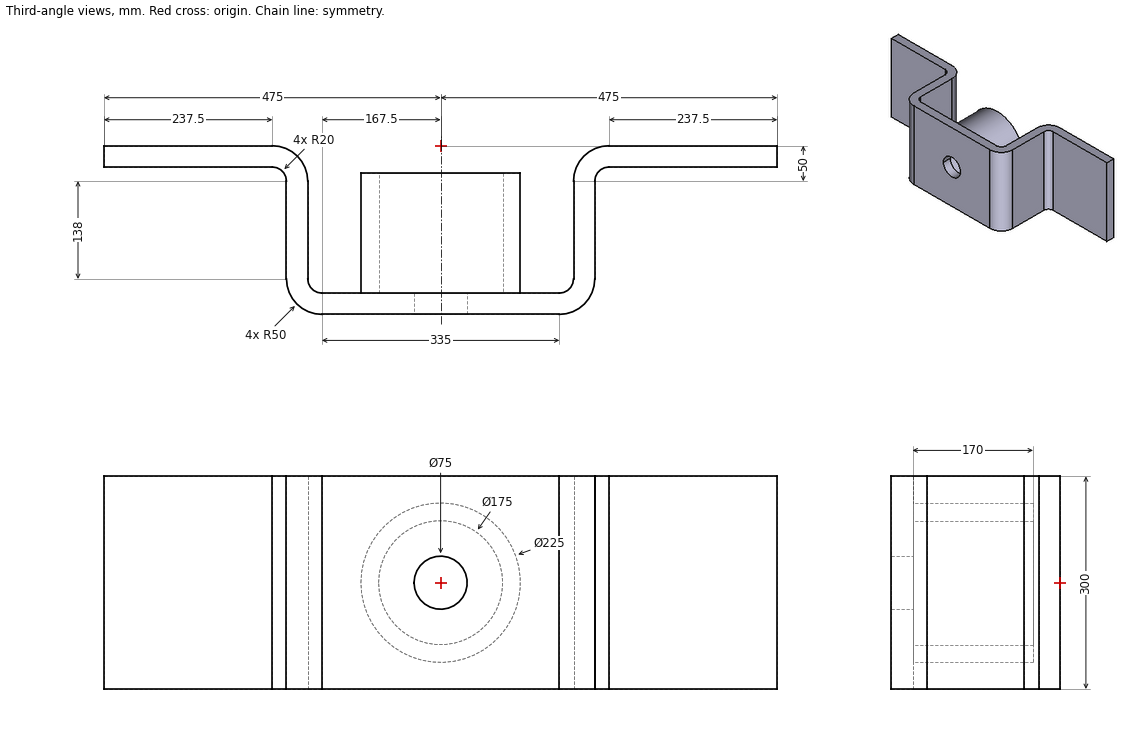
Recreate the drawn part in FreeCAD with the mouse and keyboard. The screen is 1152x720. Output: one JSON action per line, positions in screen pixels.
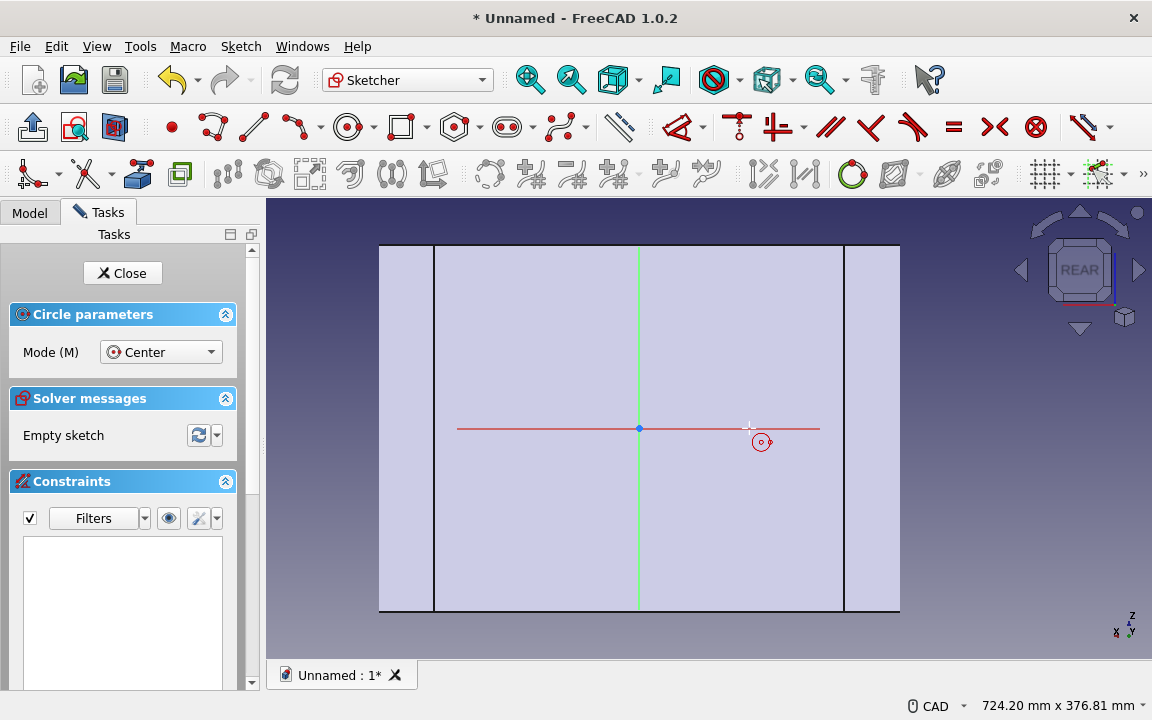
{"action": "left_click", "coordinate": [639, 428]}
{"action": "left_click", "coordinate": [737, 331]}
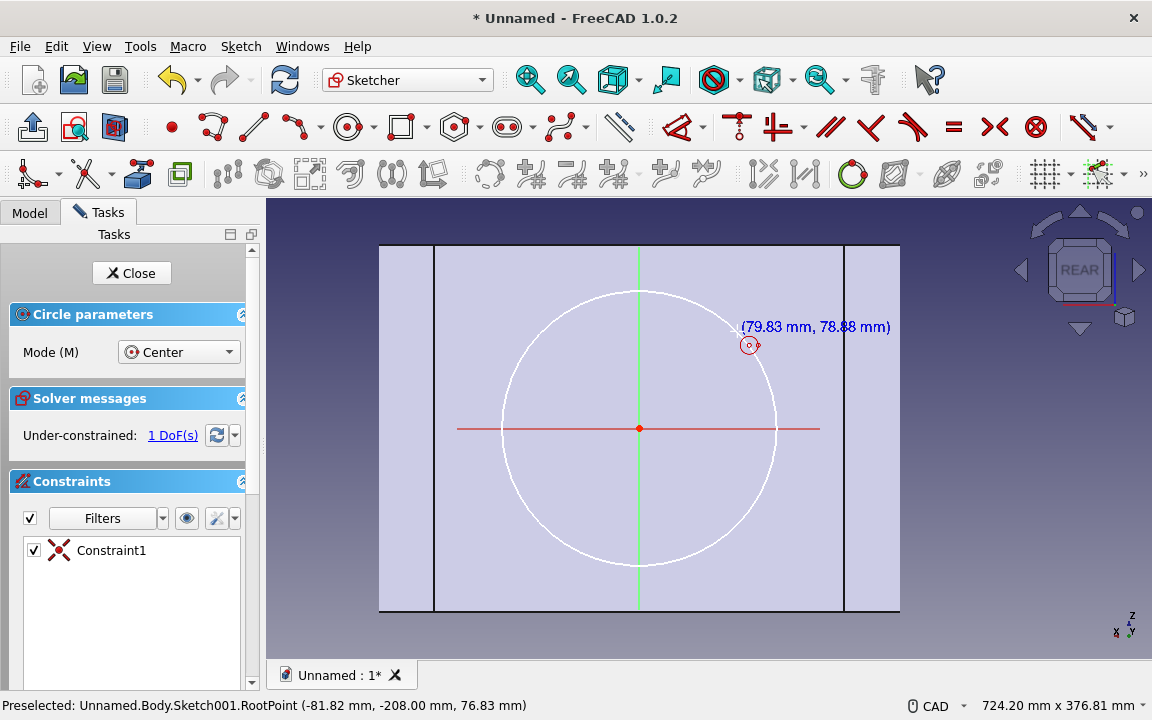
{"action": "left_click", "coordinate": [639, 428]}
{"action": "left_click", "coordinate": [715, 353]}
{"action": "key", "text": "Escape"}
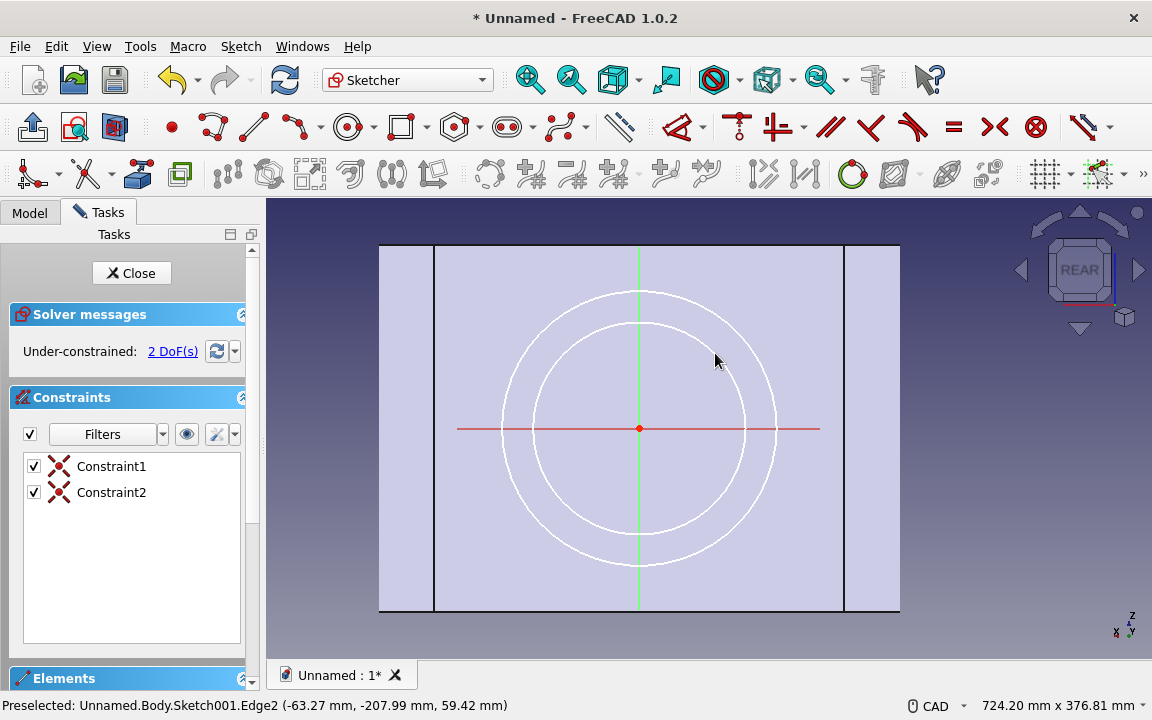
{"action": "key", "text": "d"}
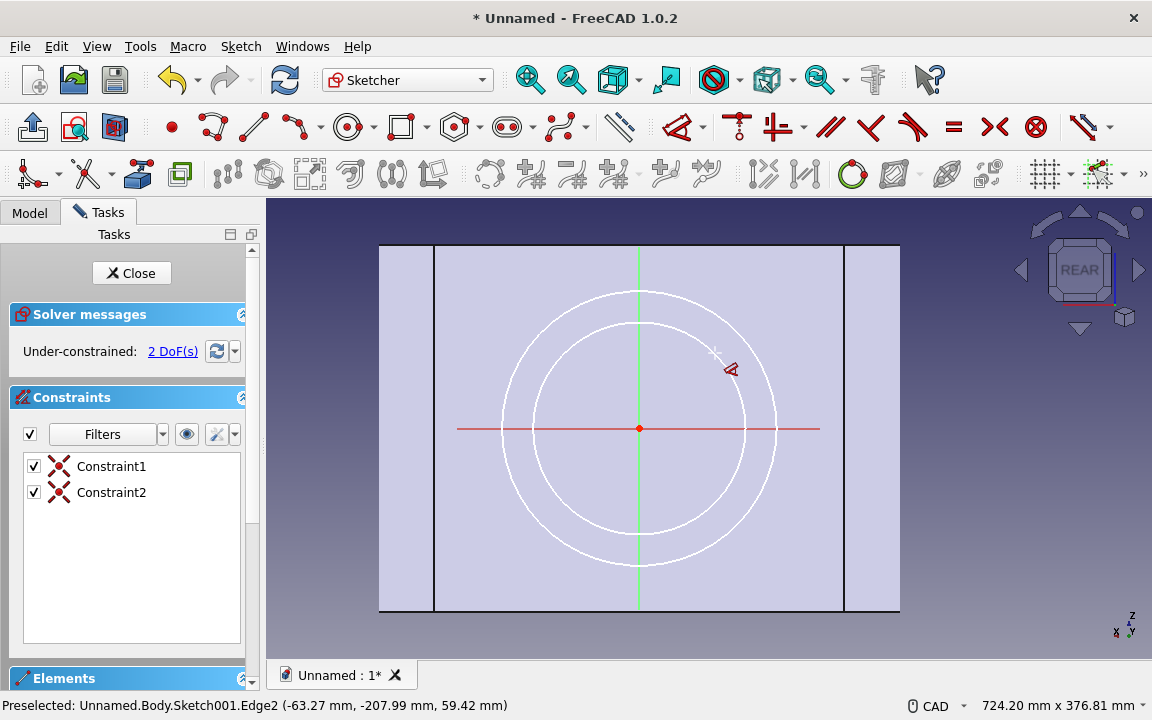
{"action": "left_click", "coordinate": [736, 331]}
{"action": "left_click", "coordinate": [759, 308]}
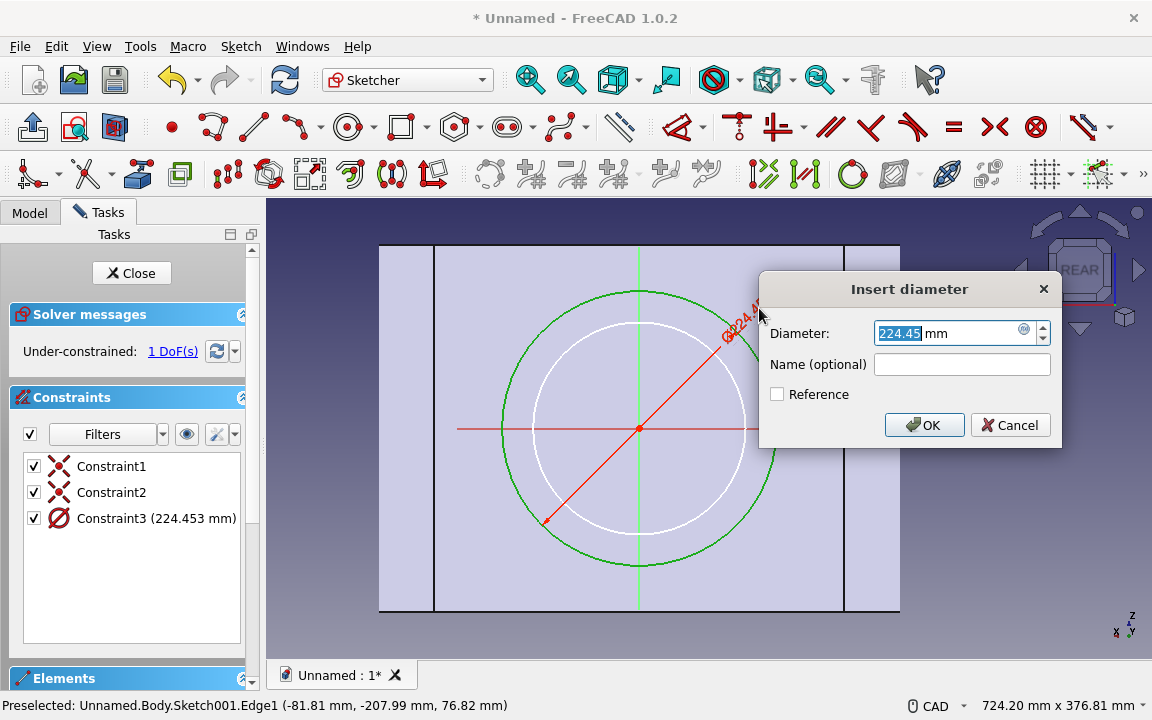
{"action": "type", "text": "225"}
{"action": "key", "text": "Return"}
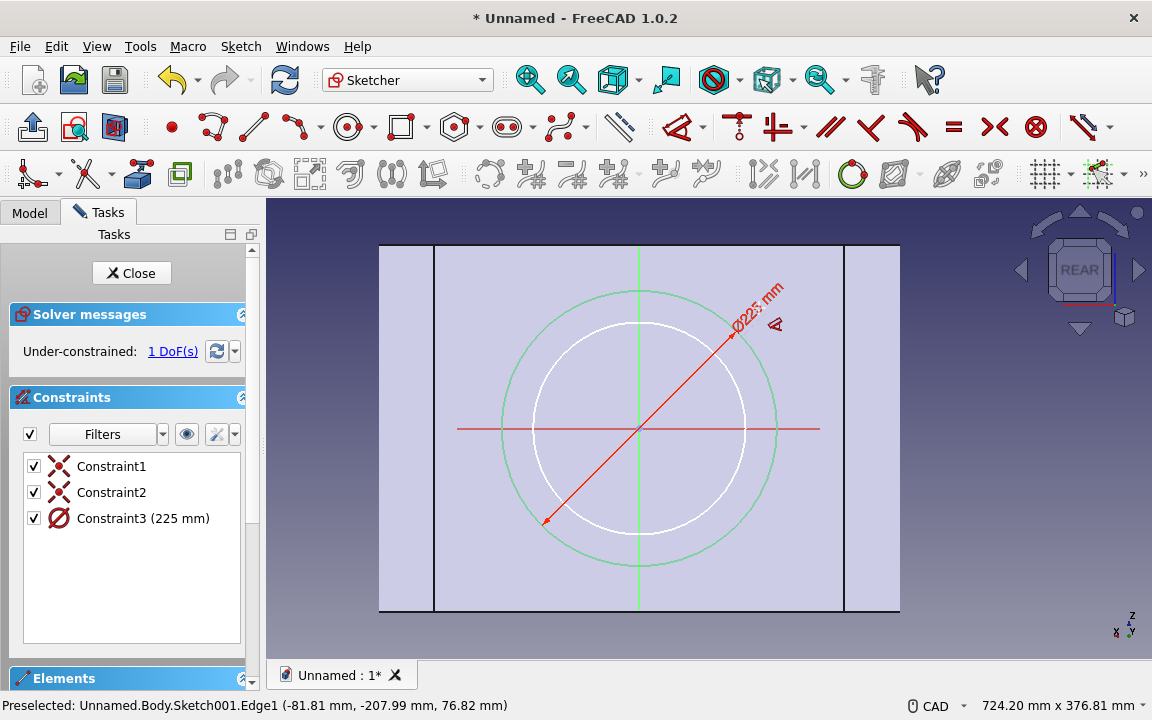
{"action": "left_click", "coordinate": [714, 353]}
{"action": "left_click", "coordinate": [794, 382]}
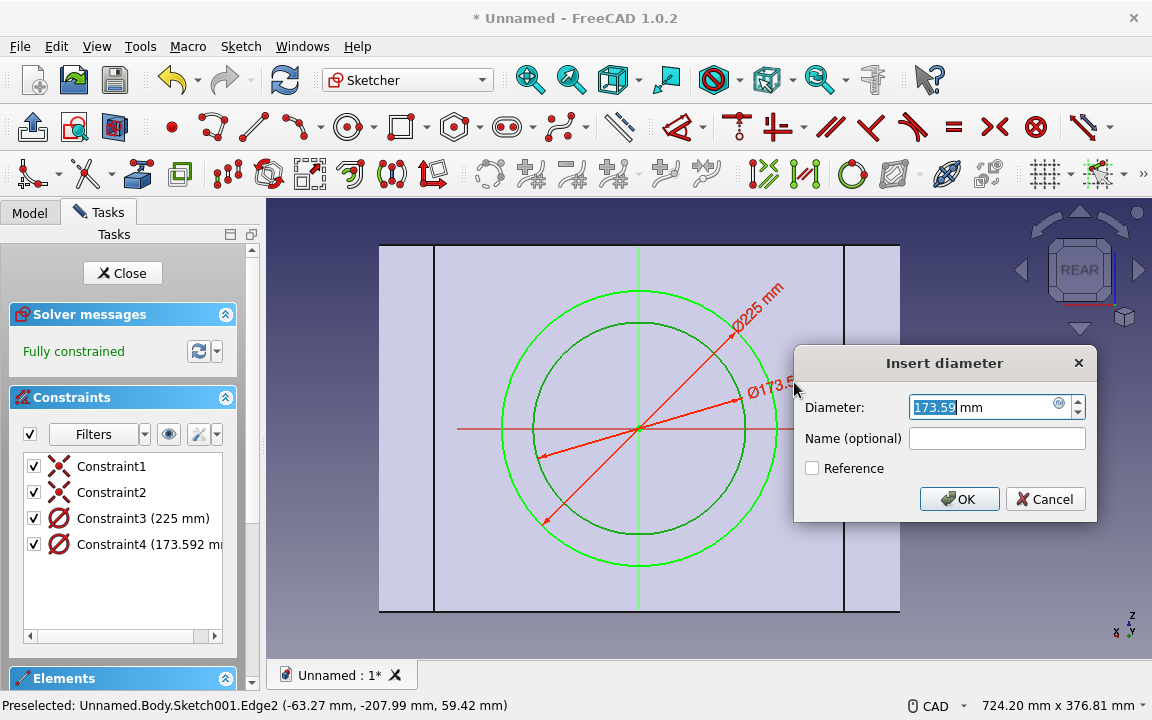
{"action": "type", "text": "175"}
{"action": "key", "text": "Return"}
{"action": "key", "text": "Escape"}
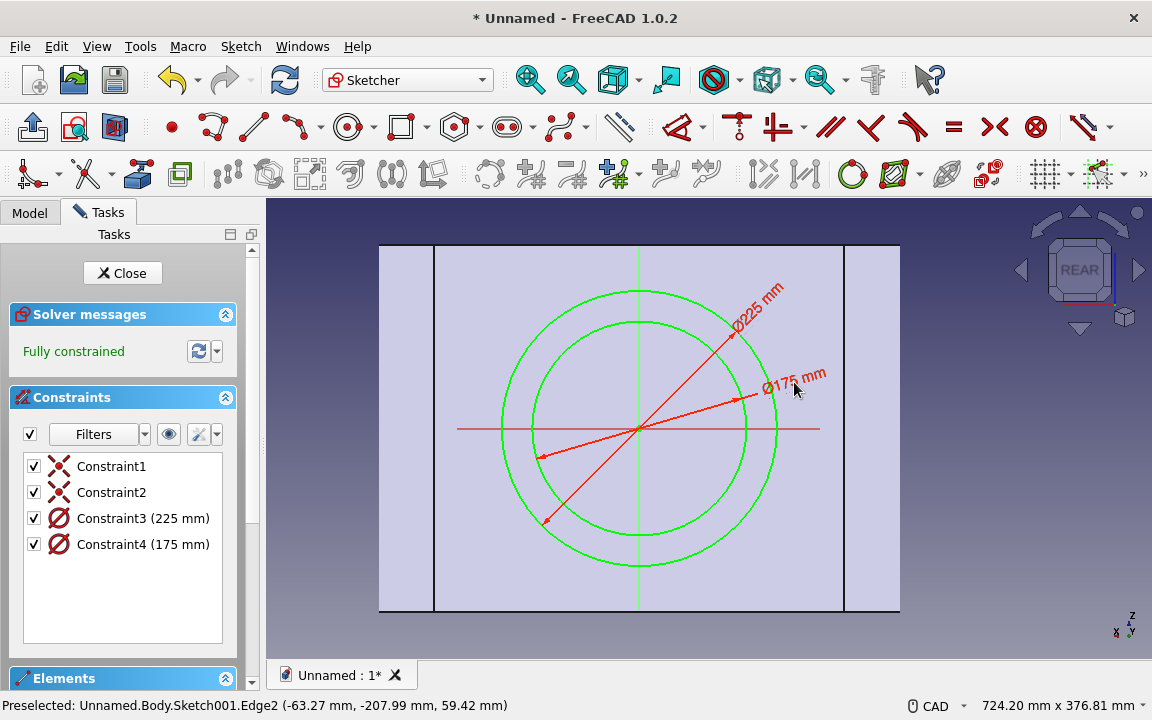
{"action": "left_click", "coordinate": [123, 273]}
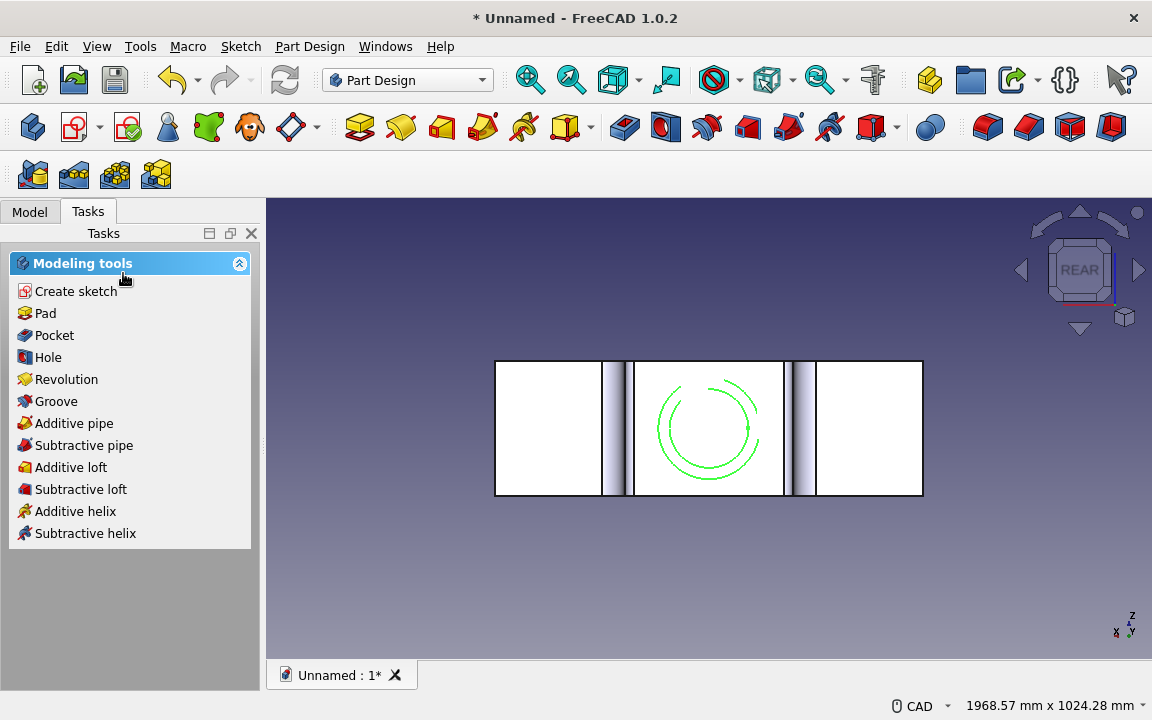
{"action": "left_click", "coordinate": [360, 128]}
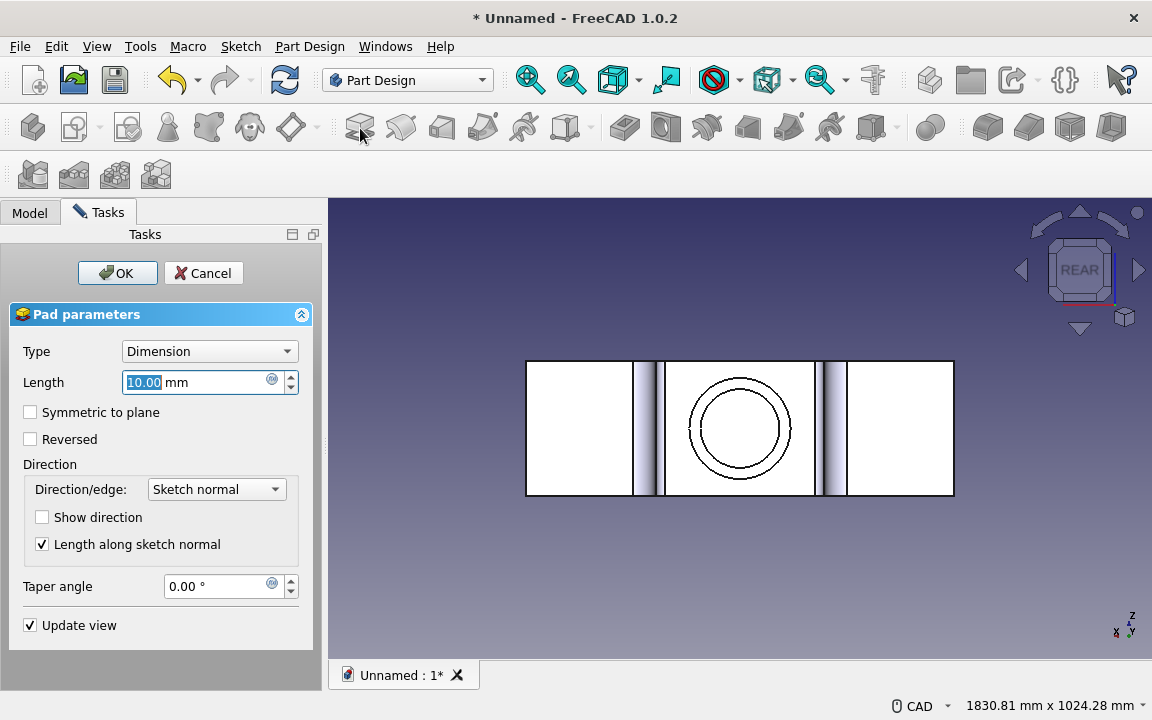
{"action": "type", "text": "170"}
{"action": "key", "text": "Tab"}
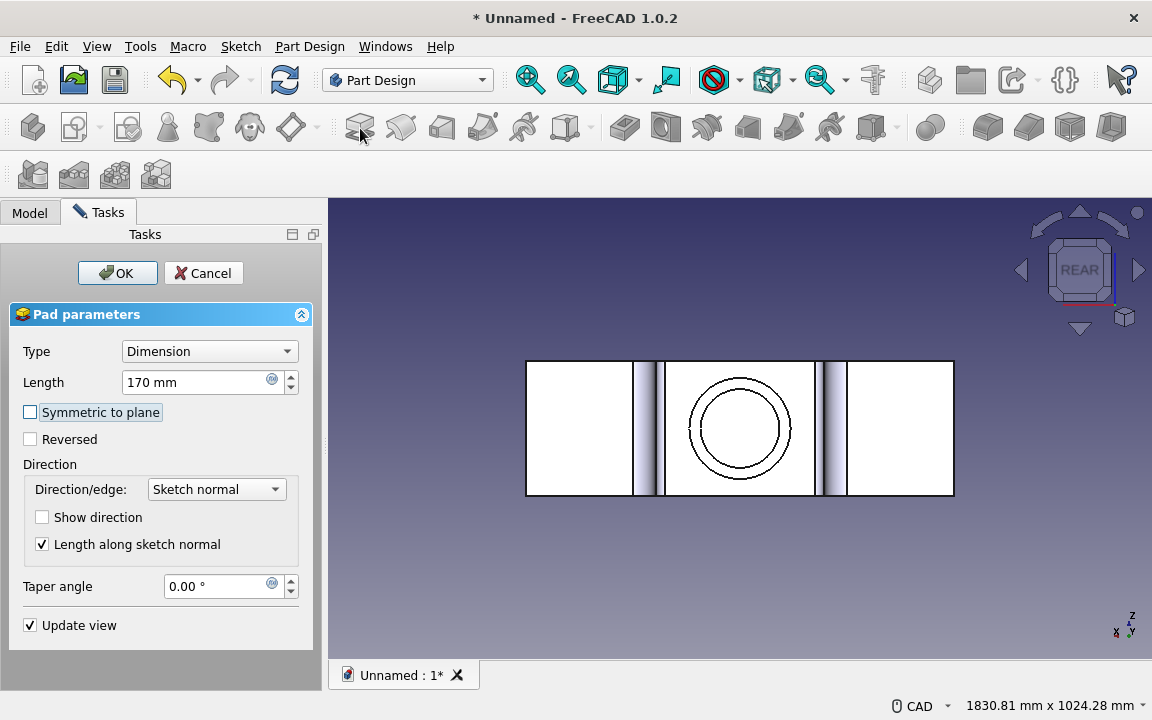
{"action": "left_click", "coordinate": [118, 273]}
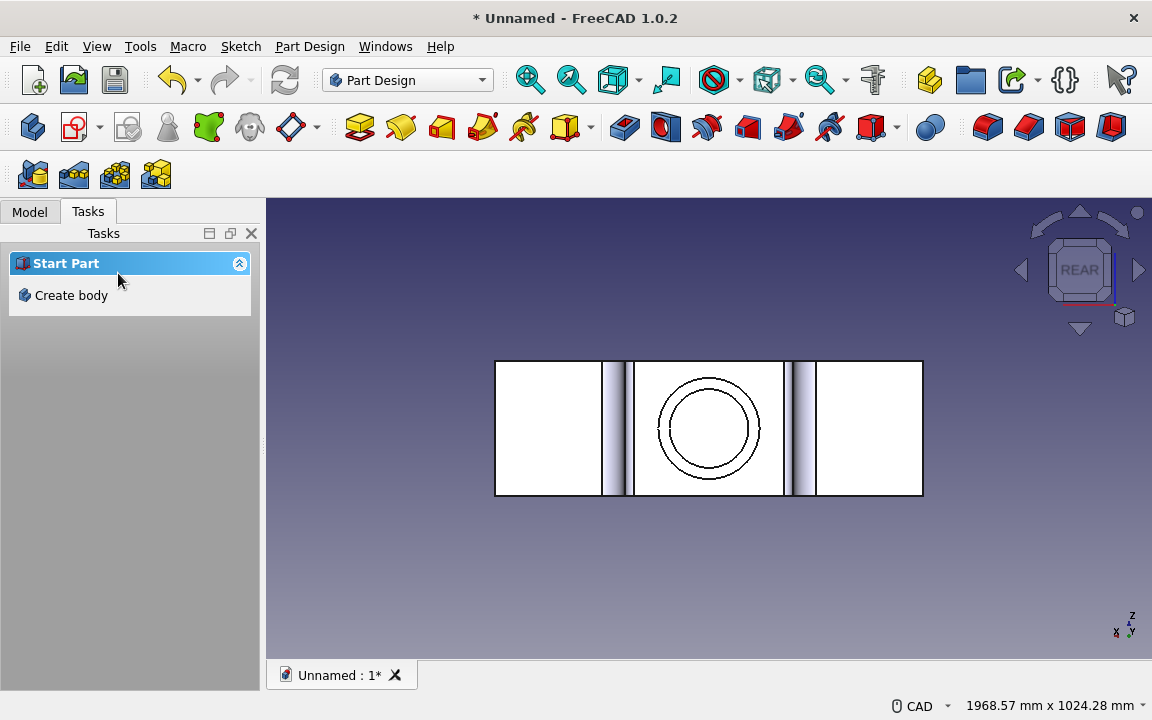
{"action": "left_click", "coordinate": [774, 389]}